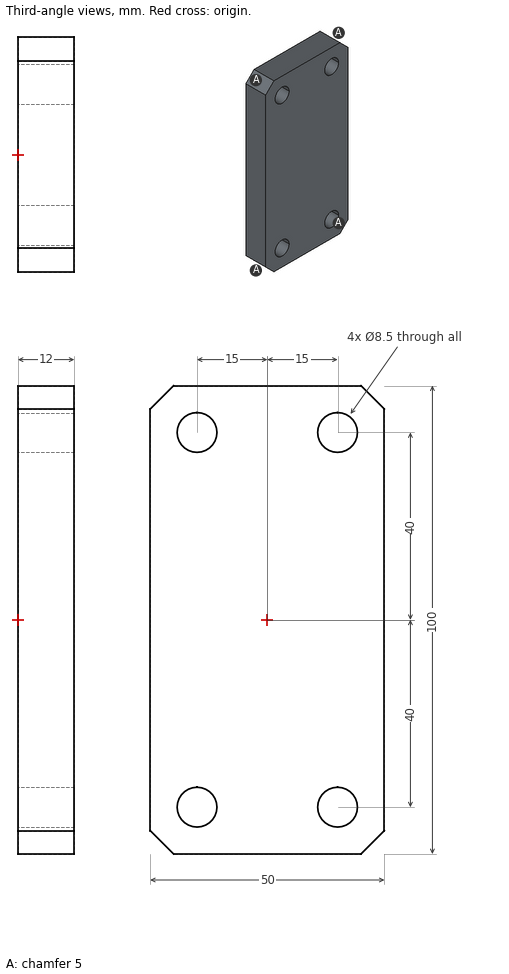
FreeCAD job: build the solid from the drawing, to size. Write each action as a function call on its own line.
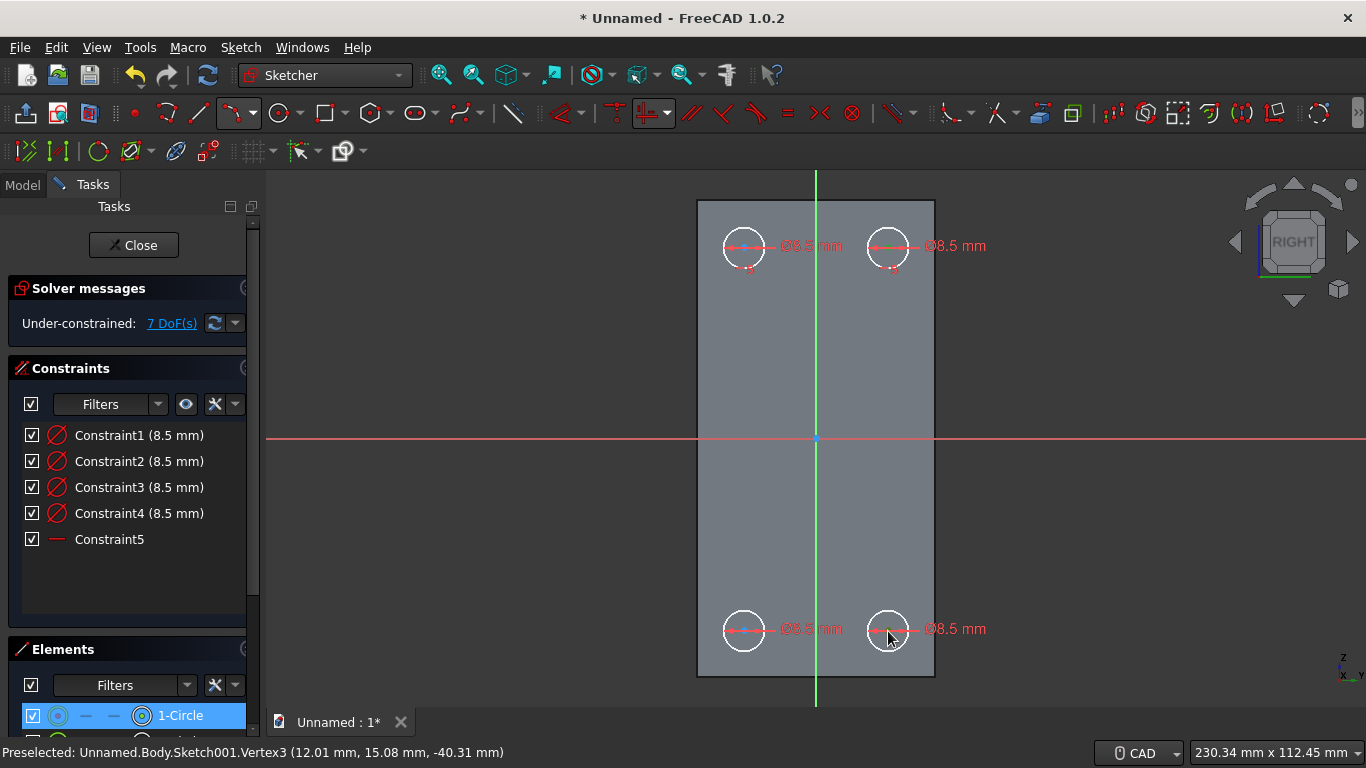
key(v)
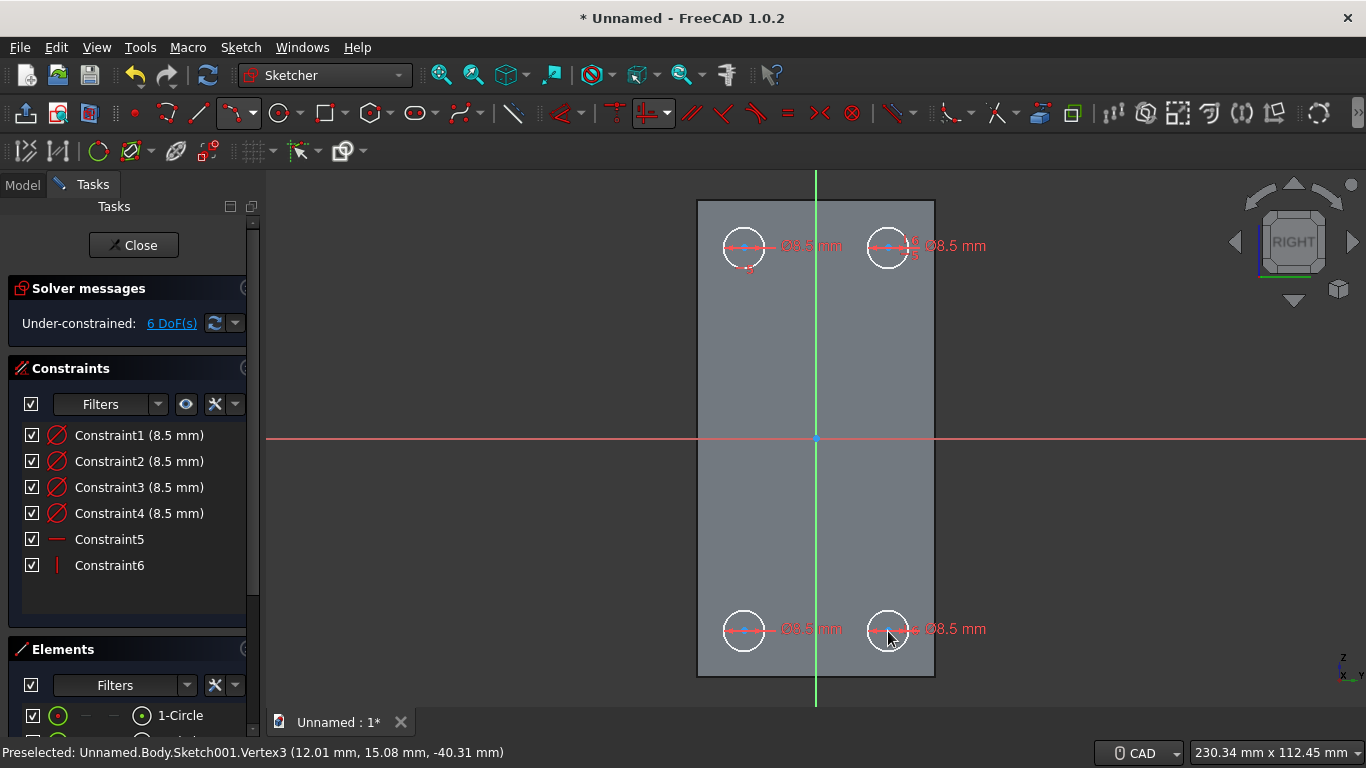
click(744, 248)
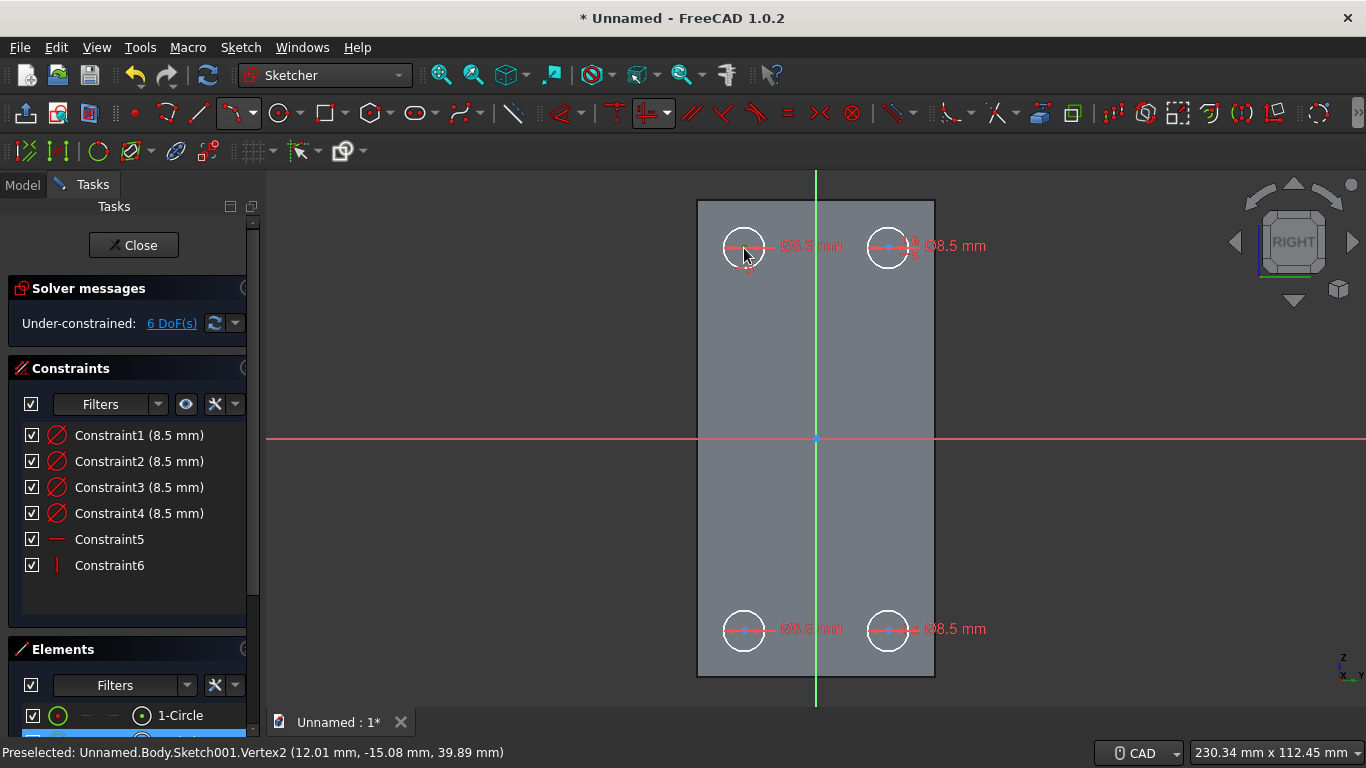
click(744, 631)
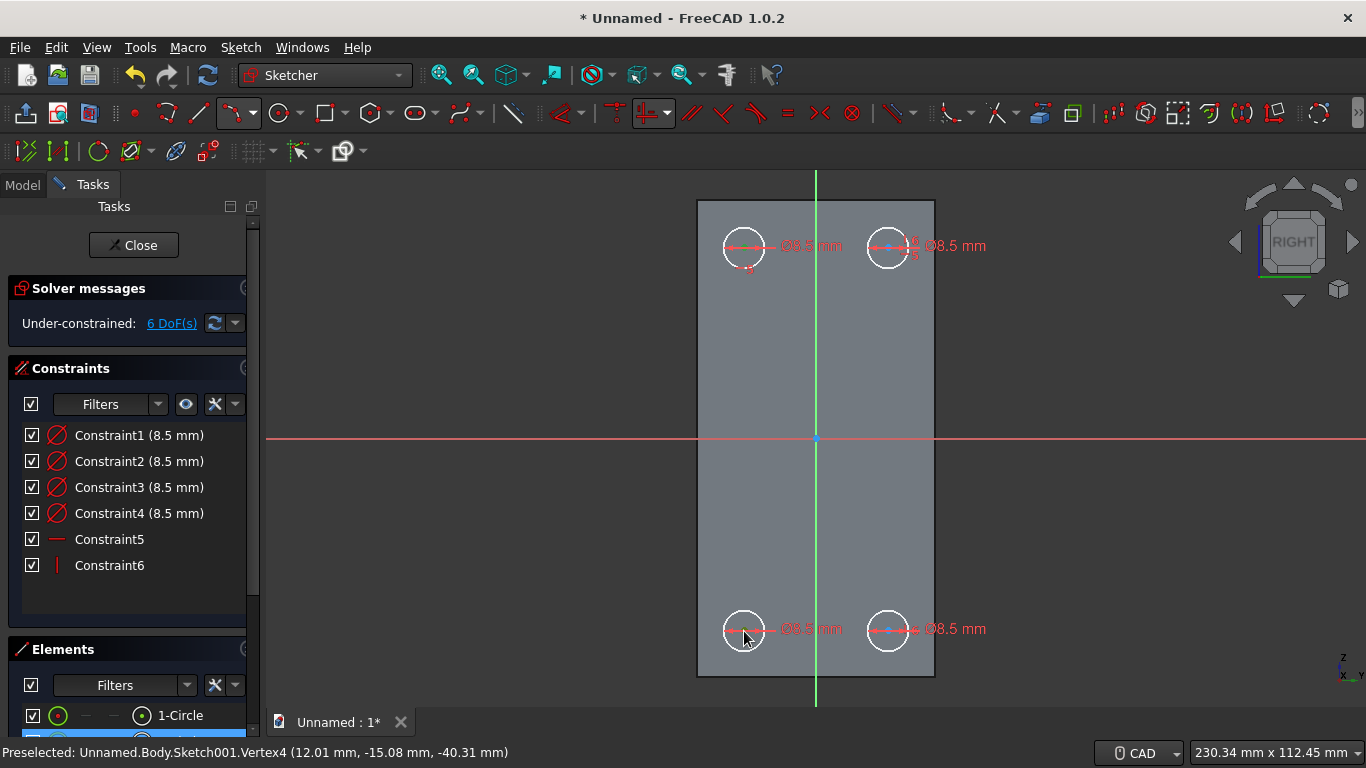
click(670, 114)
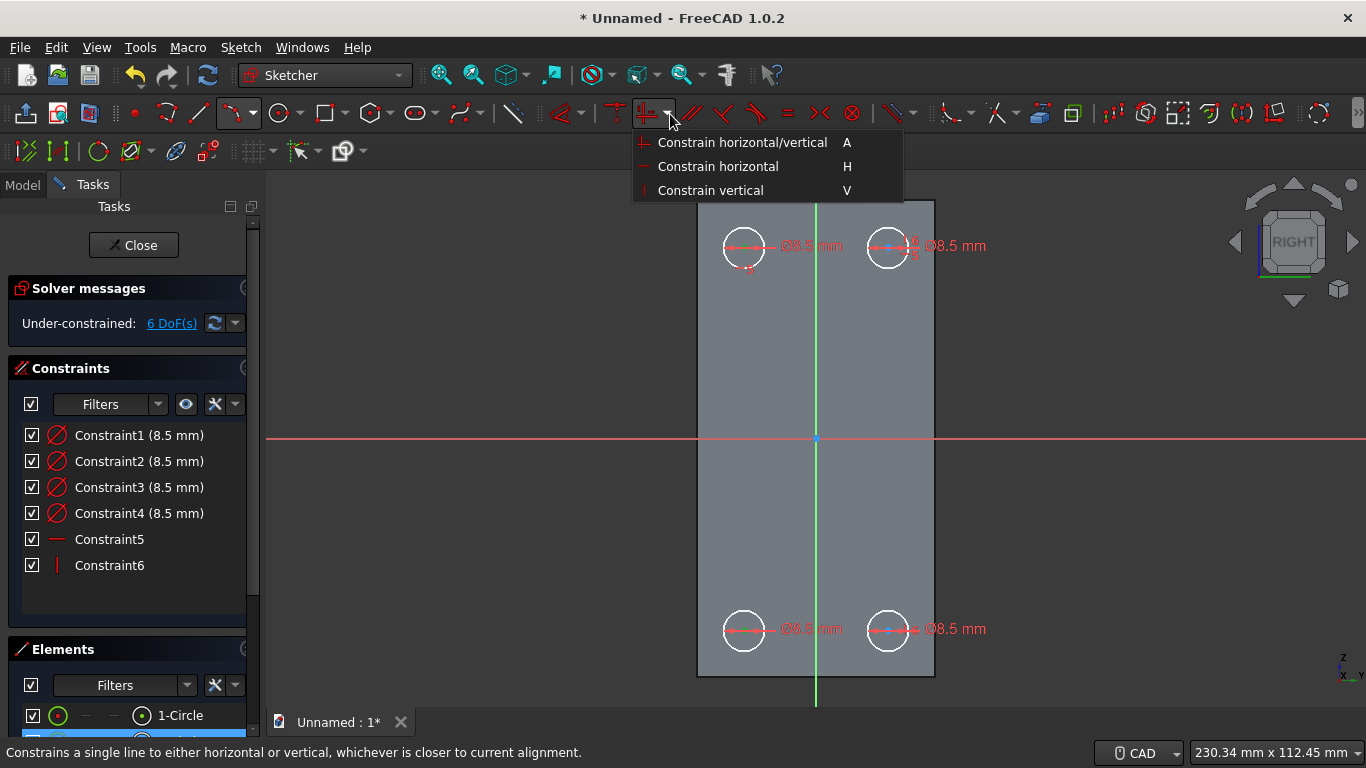
click(768, 190)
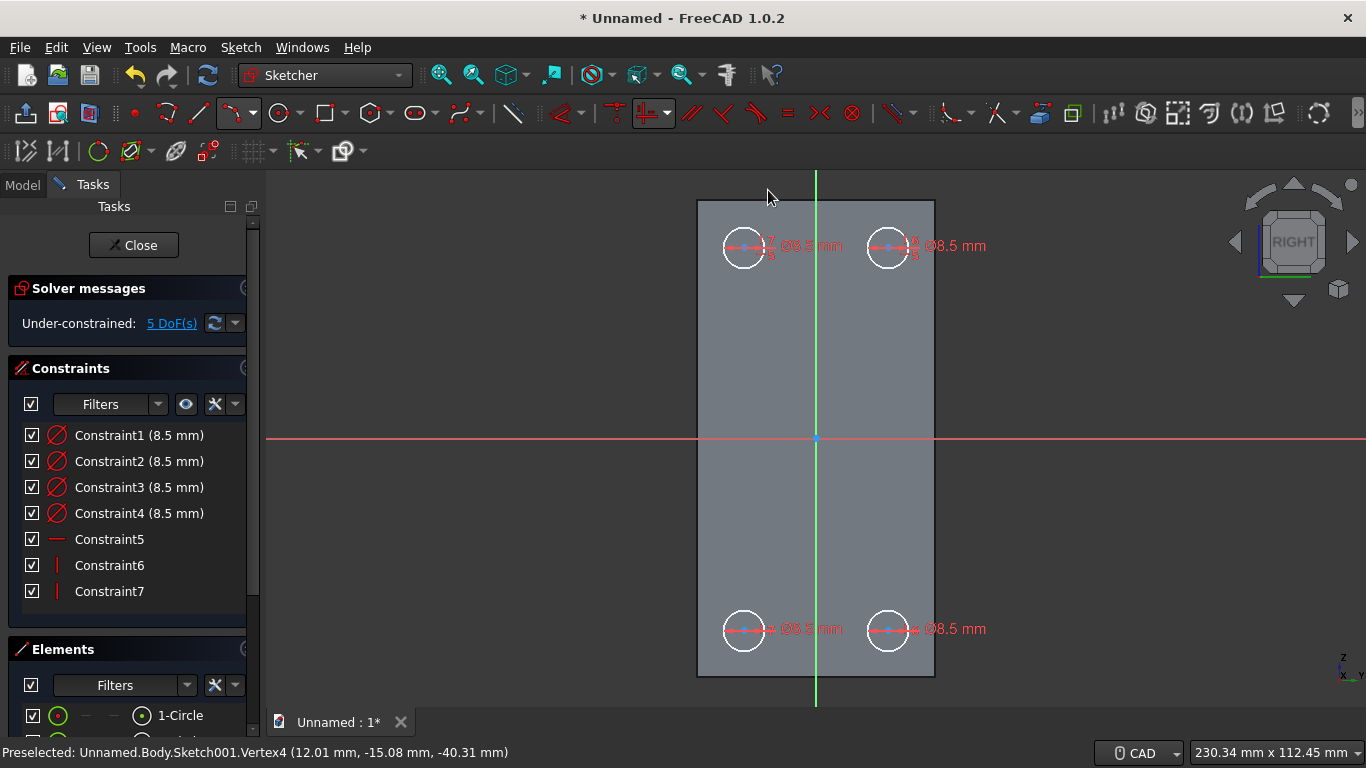
click(888, 631)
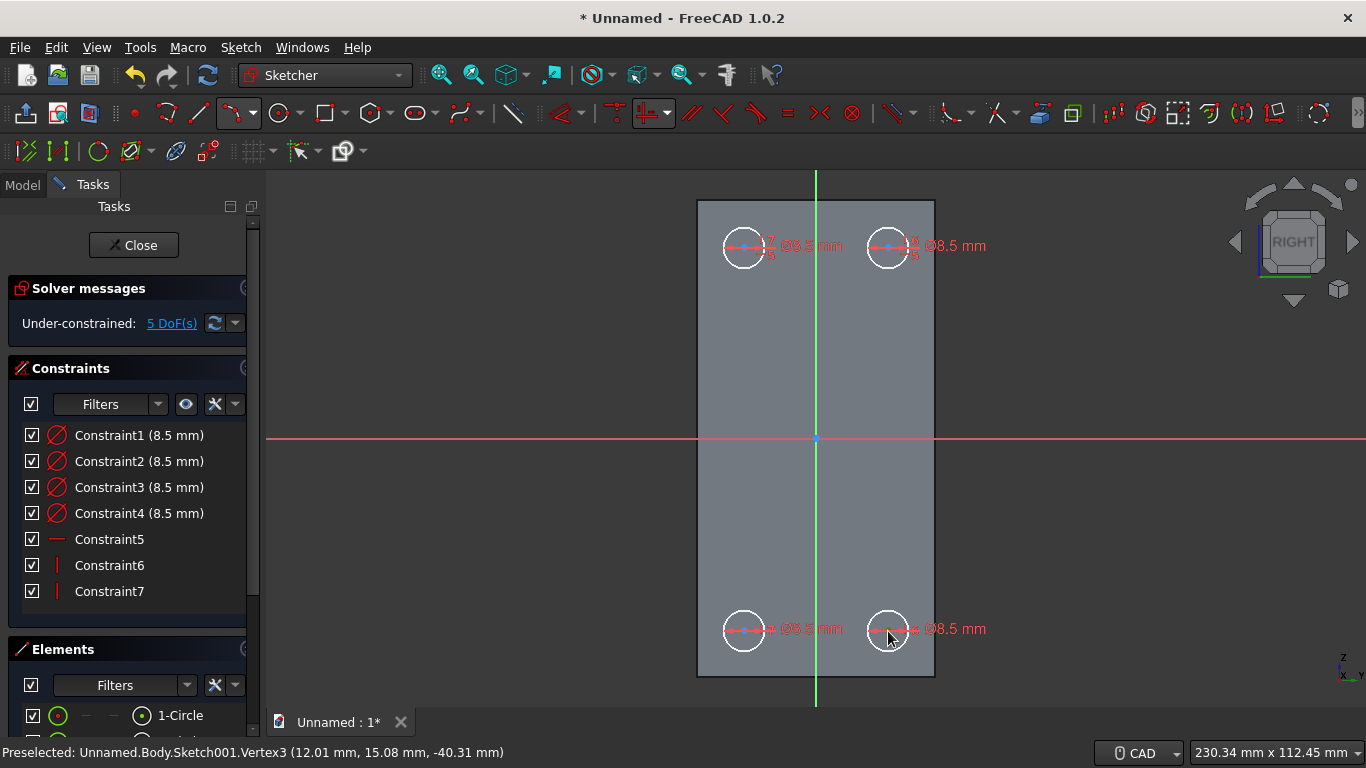
click(744, 631)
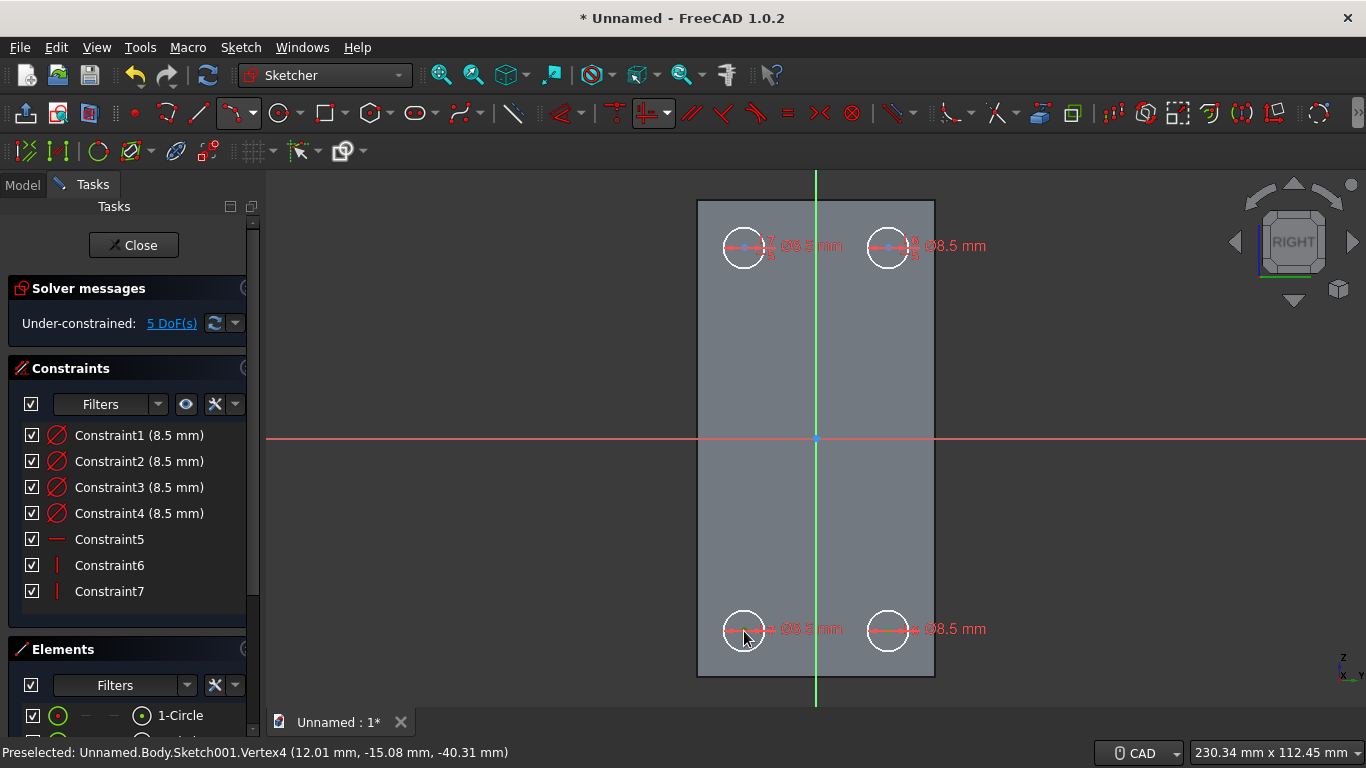
key(h)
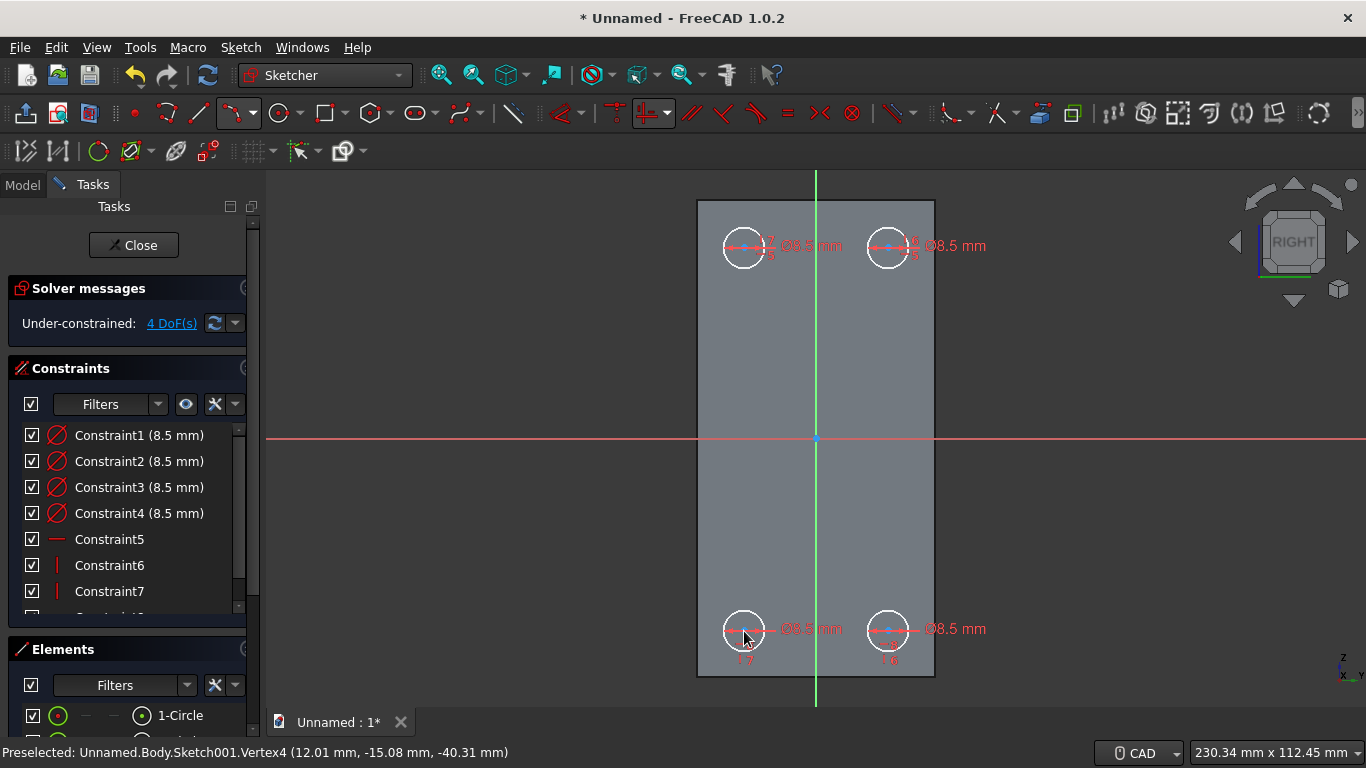
click(560, 114)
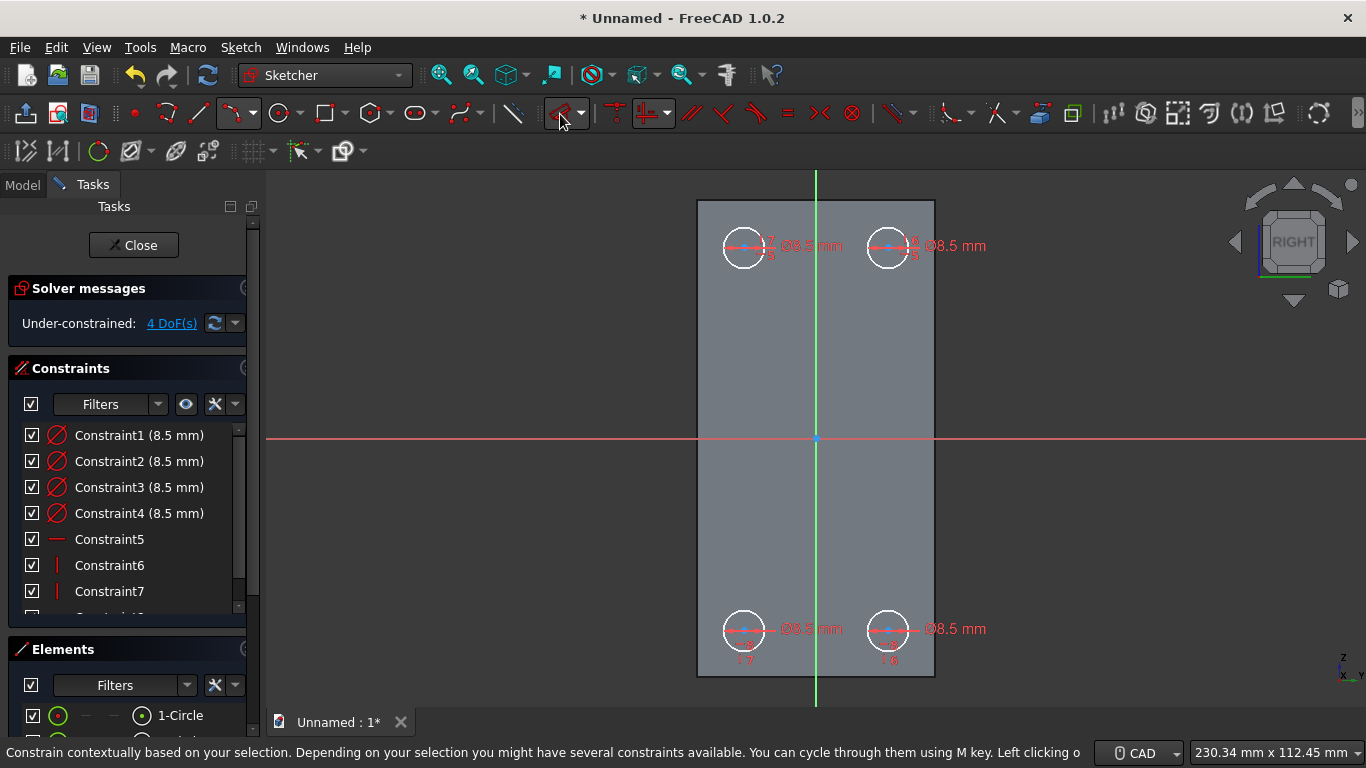
click(888, 248)
click(852, 214)